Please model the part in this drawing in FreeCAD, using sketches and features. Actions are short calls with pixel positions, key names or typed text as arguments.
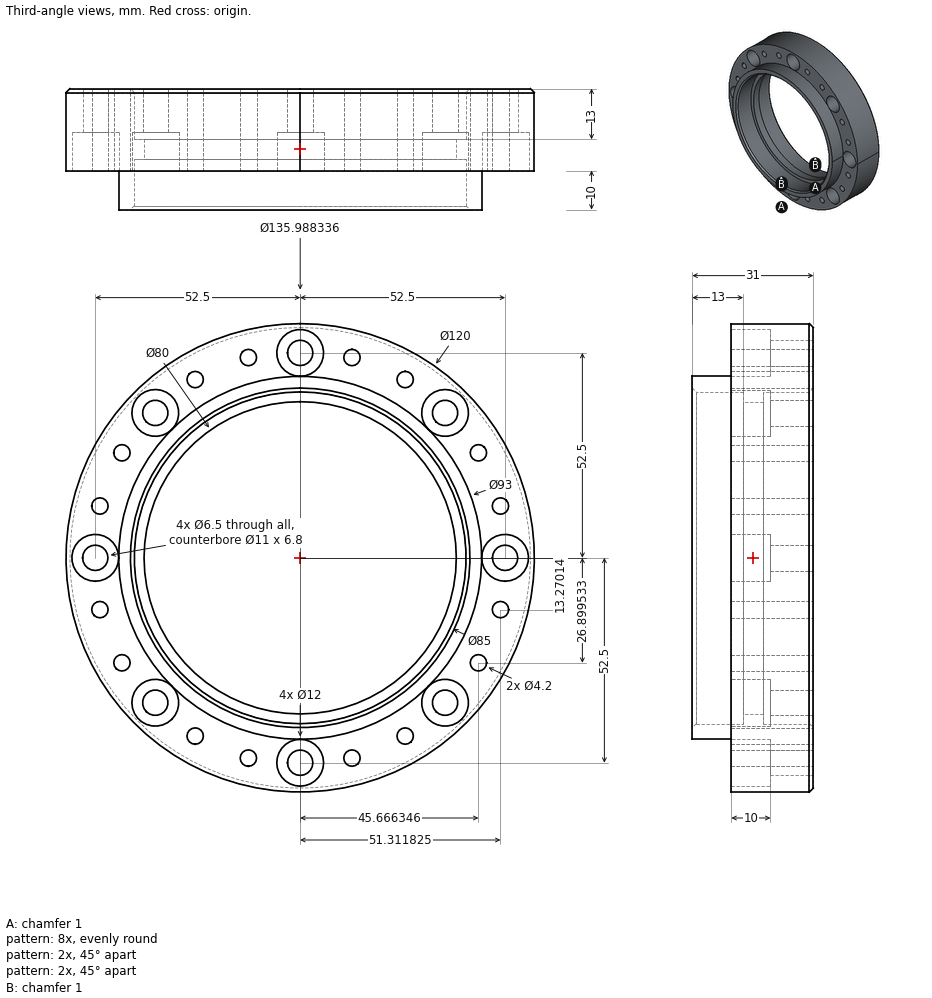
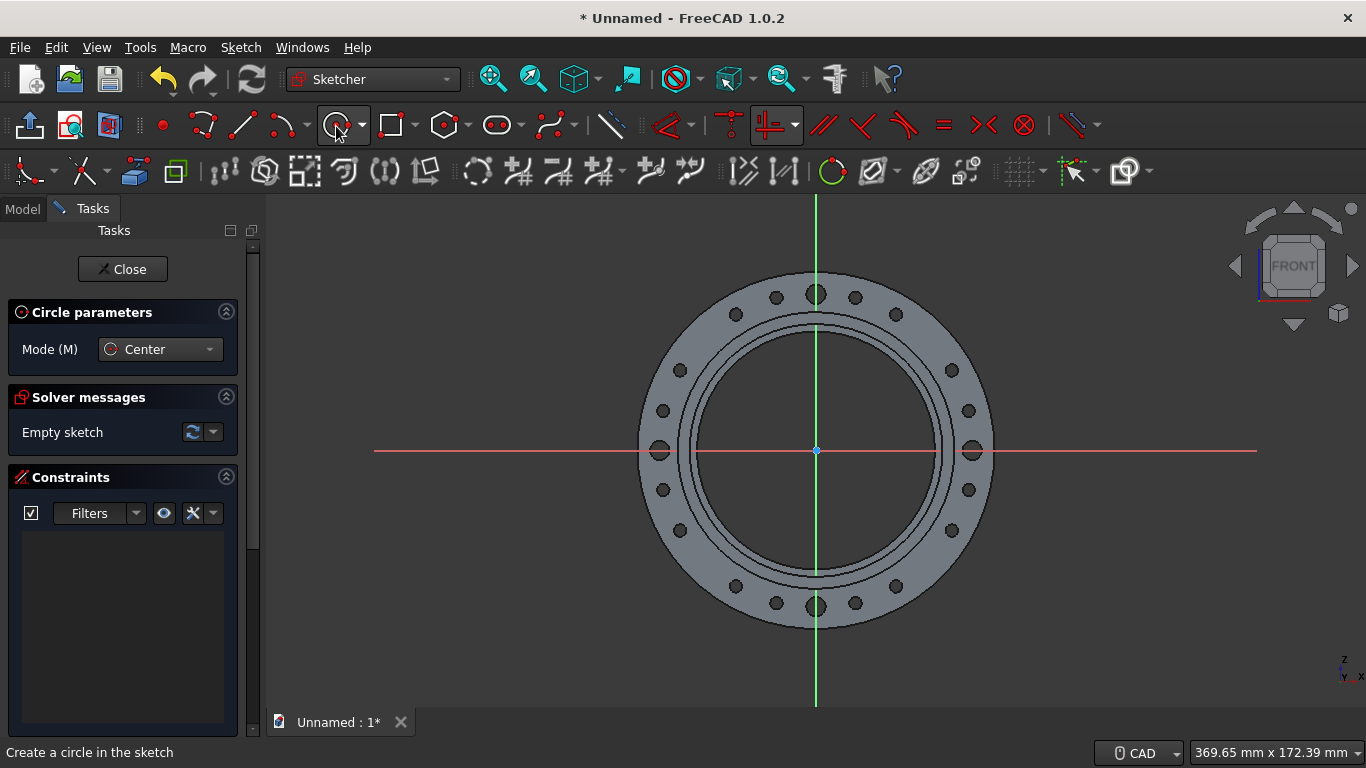
scroll(816, 607, up, 2)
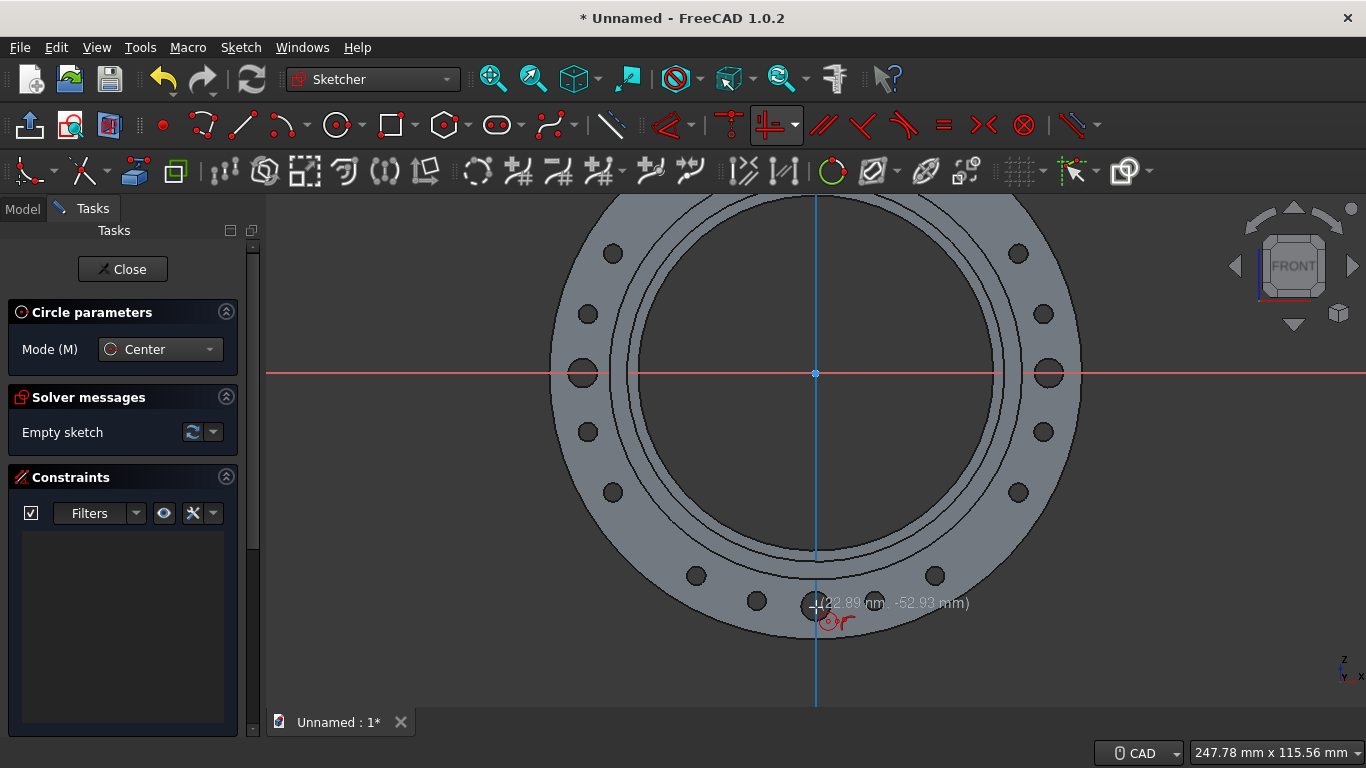
click(816, 606)
move(835, 587)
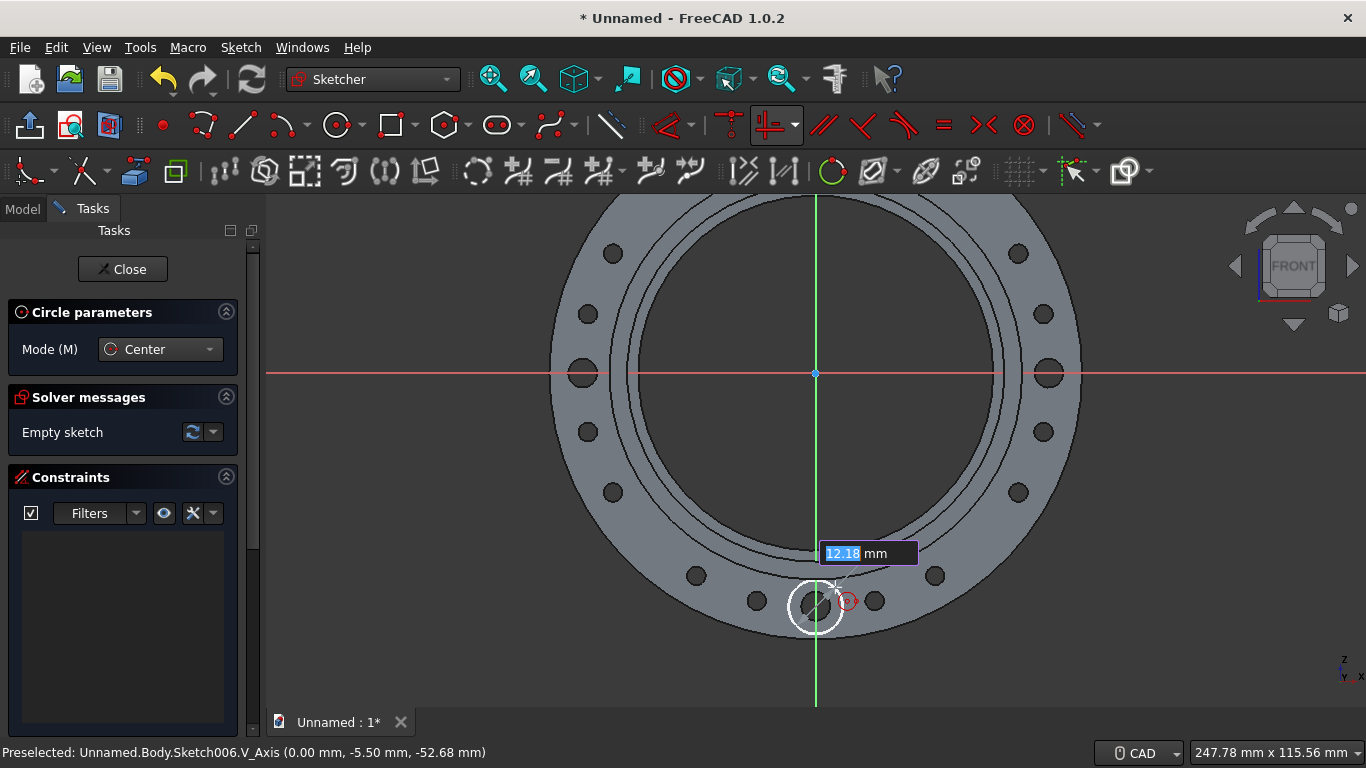
text(12)
key(Return)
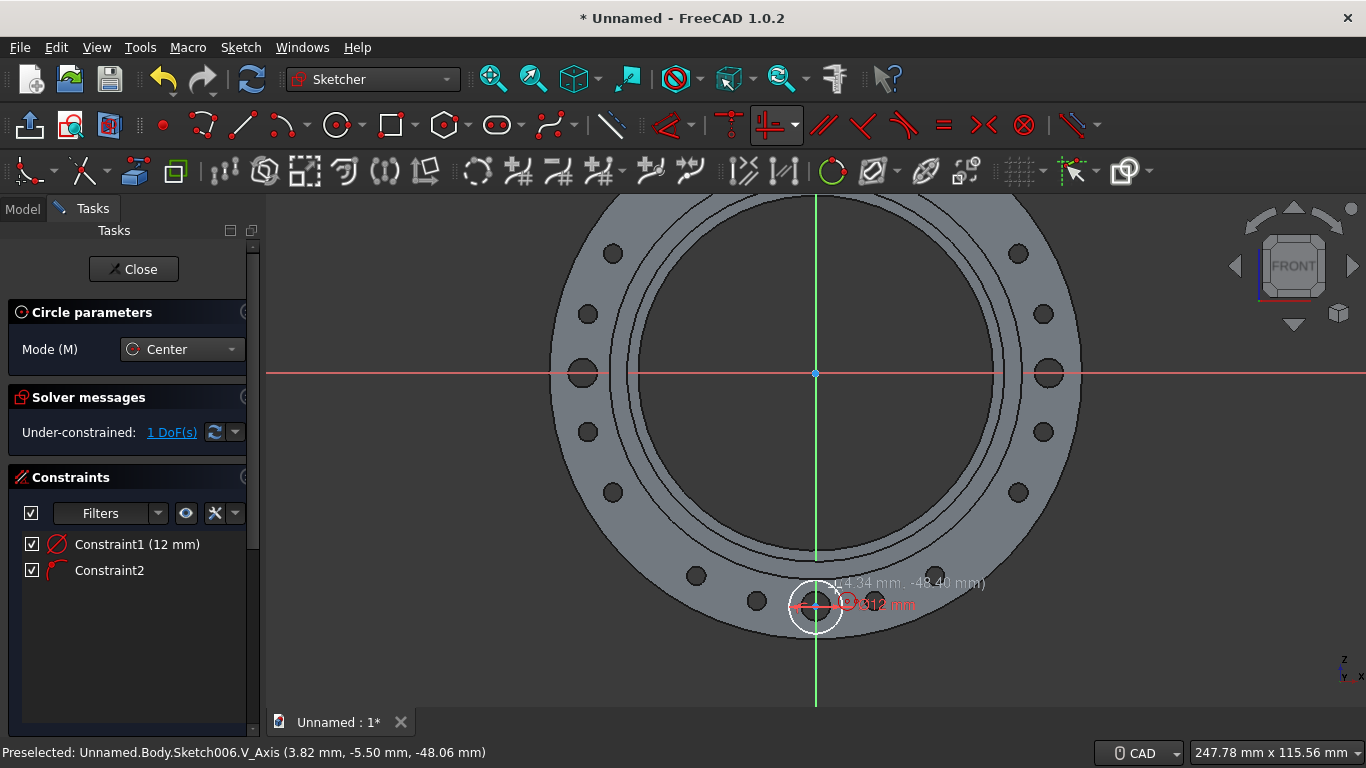
click(1049, 373)
move(1068, 354)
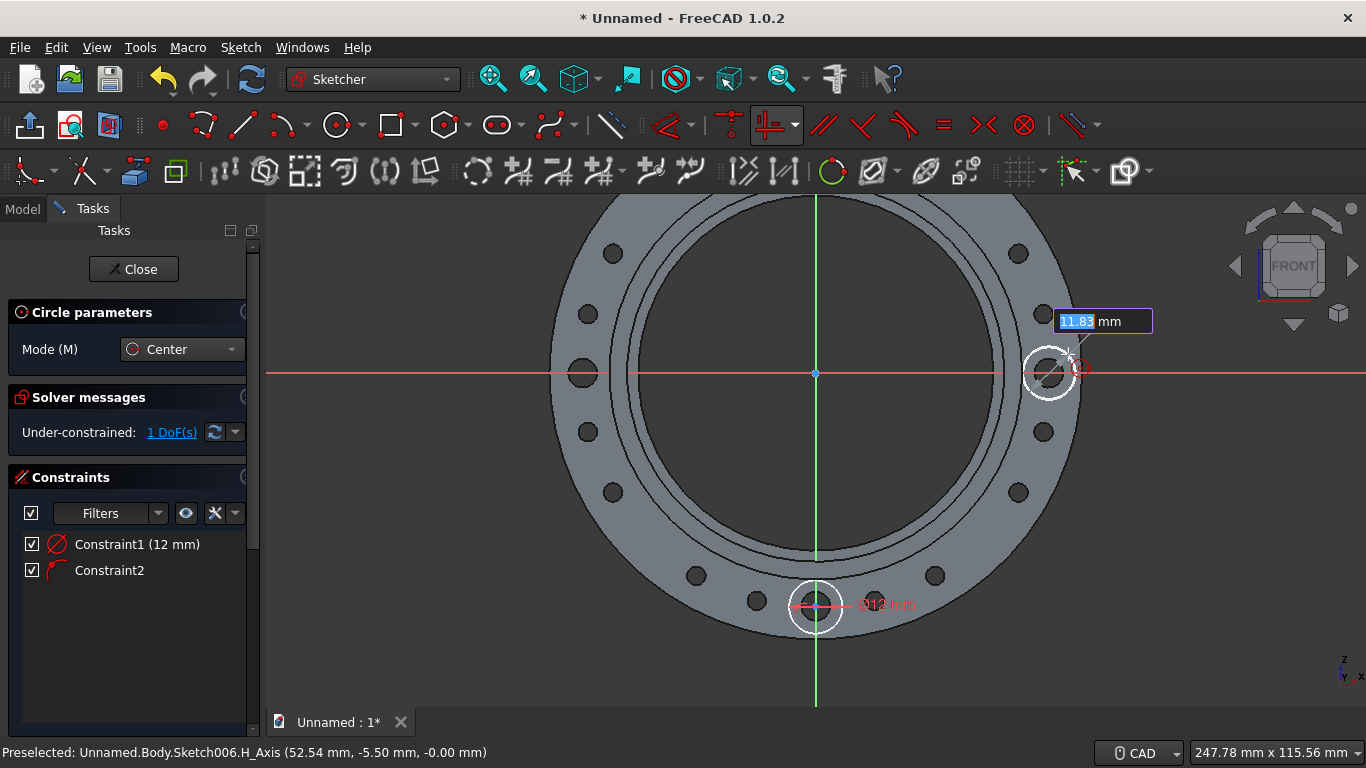
text(12)
key(Return)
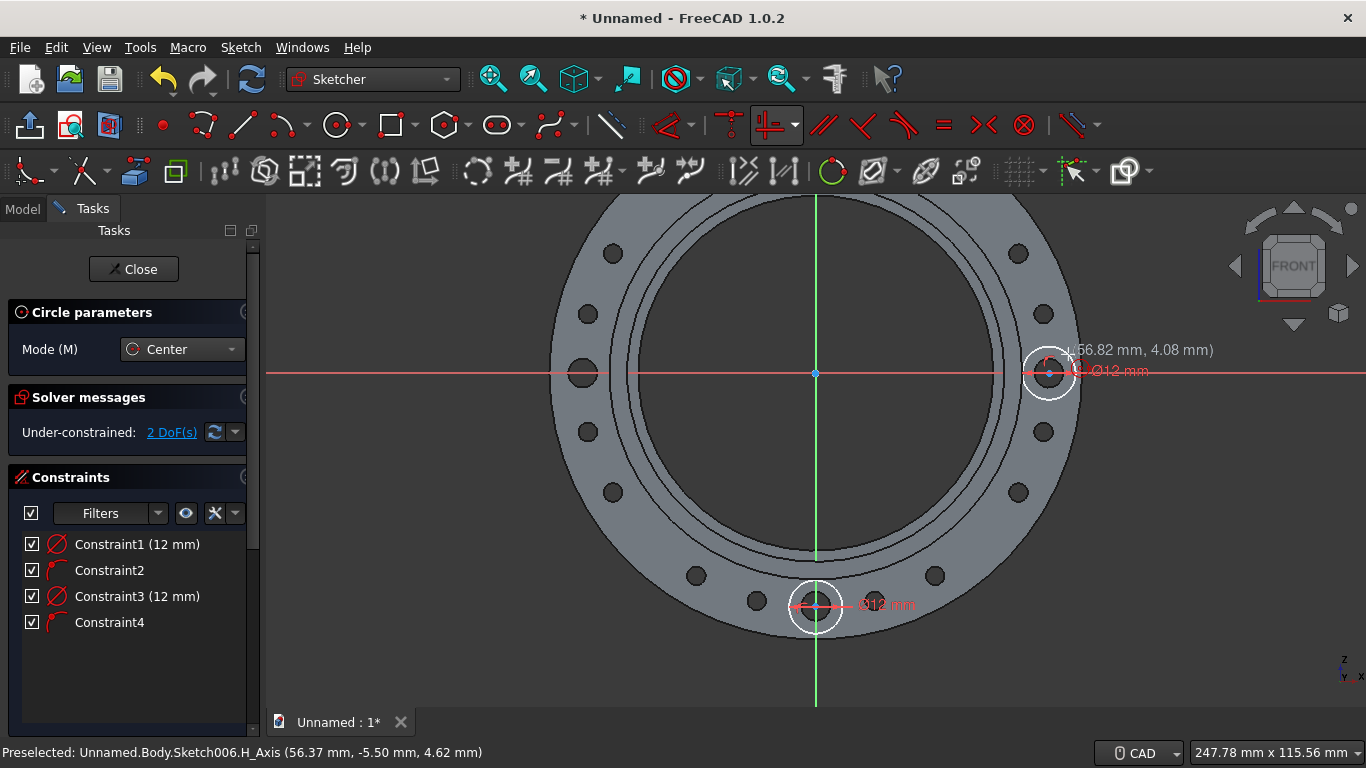
scroll(609, 608, down, 2)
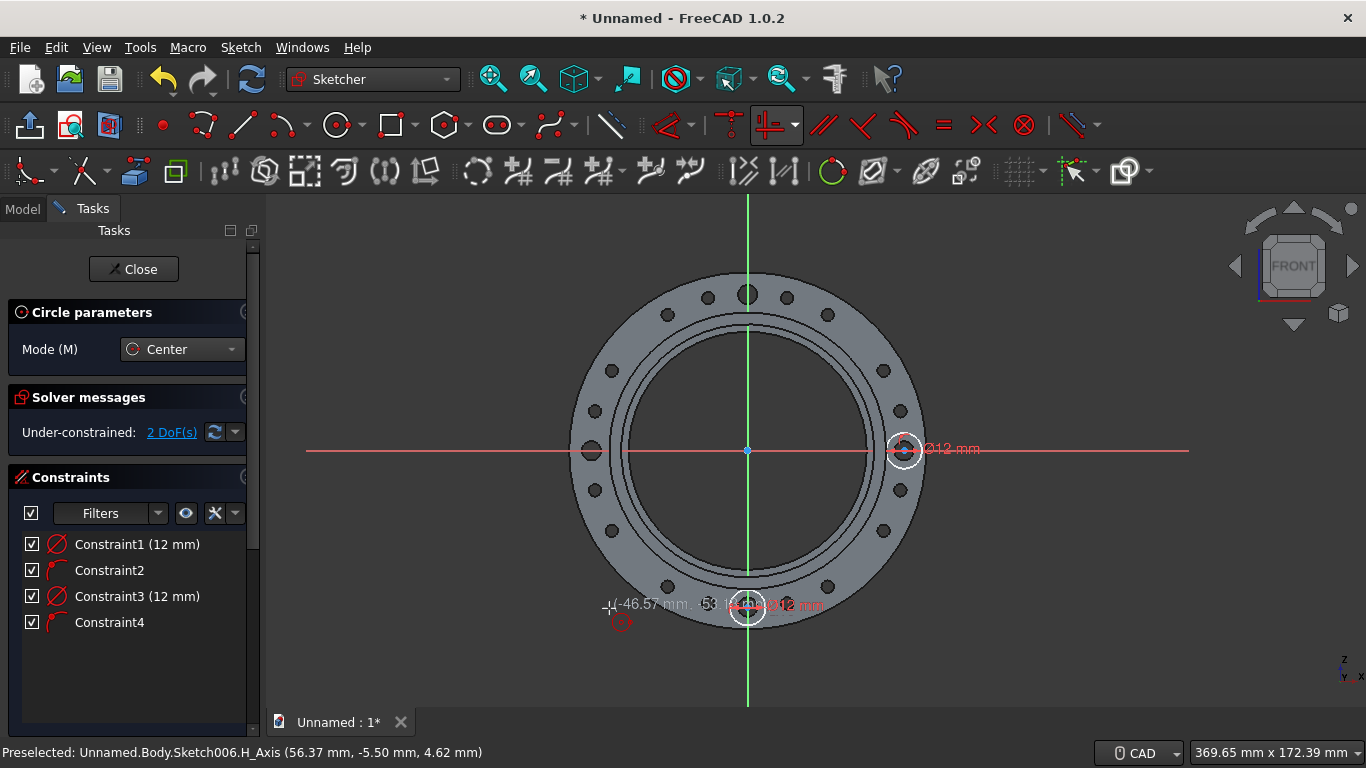
scroll(748, 295, up, 2)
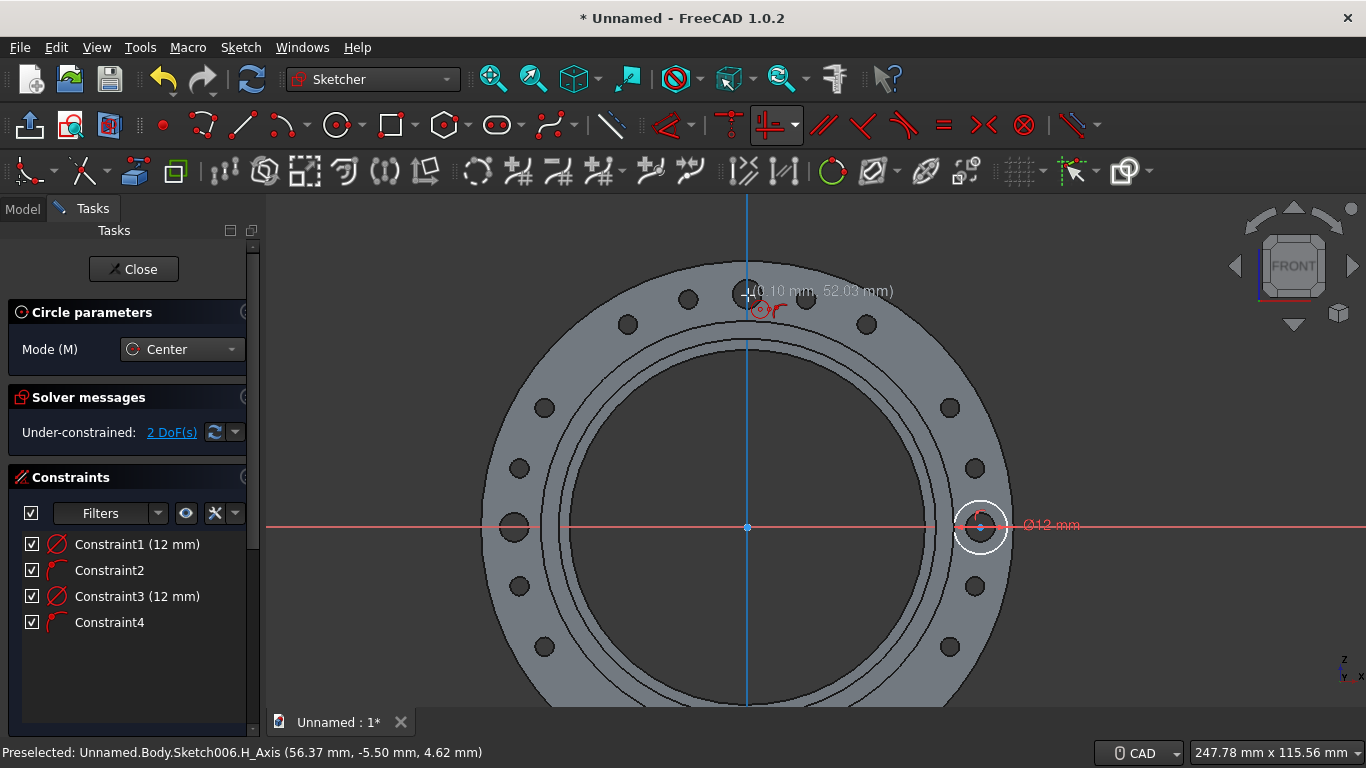
click(747, 294)
move(766, 275)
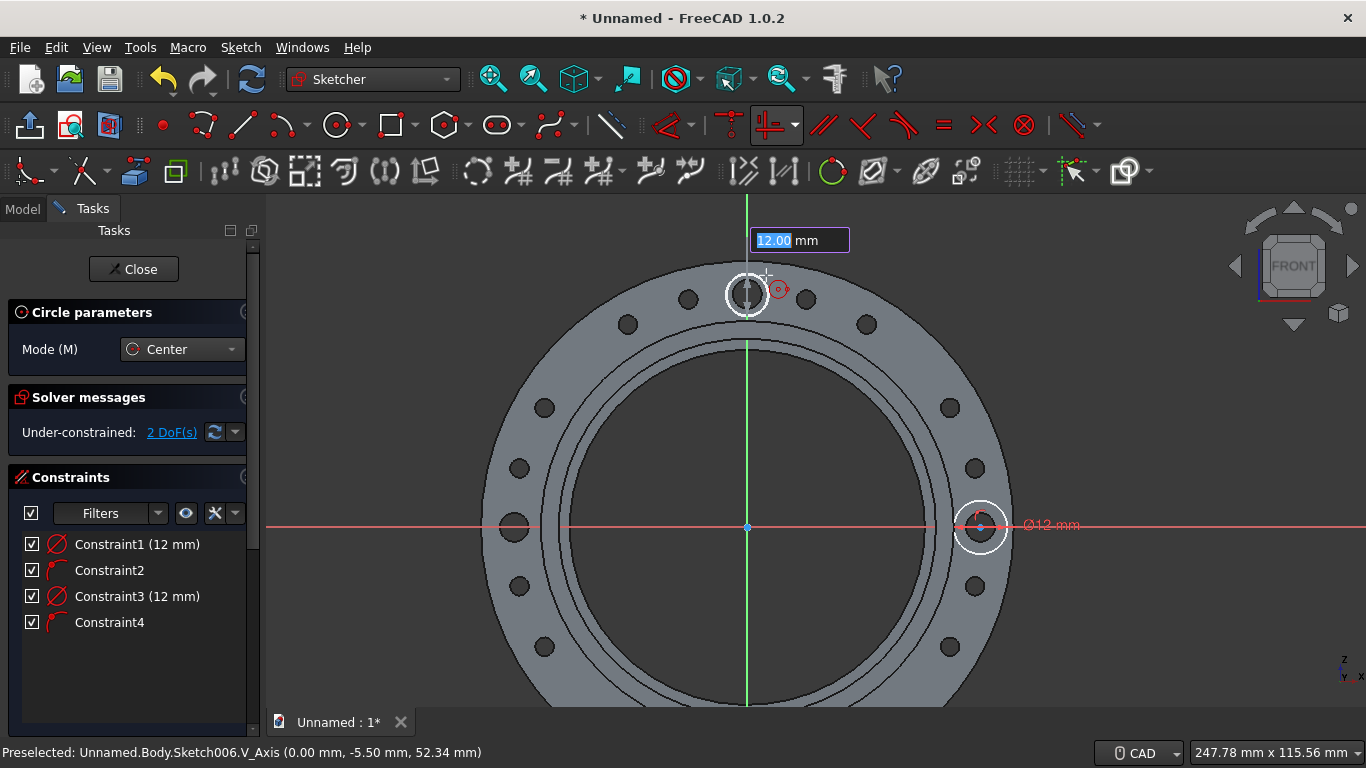
text(12)
key(Return)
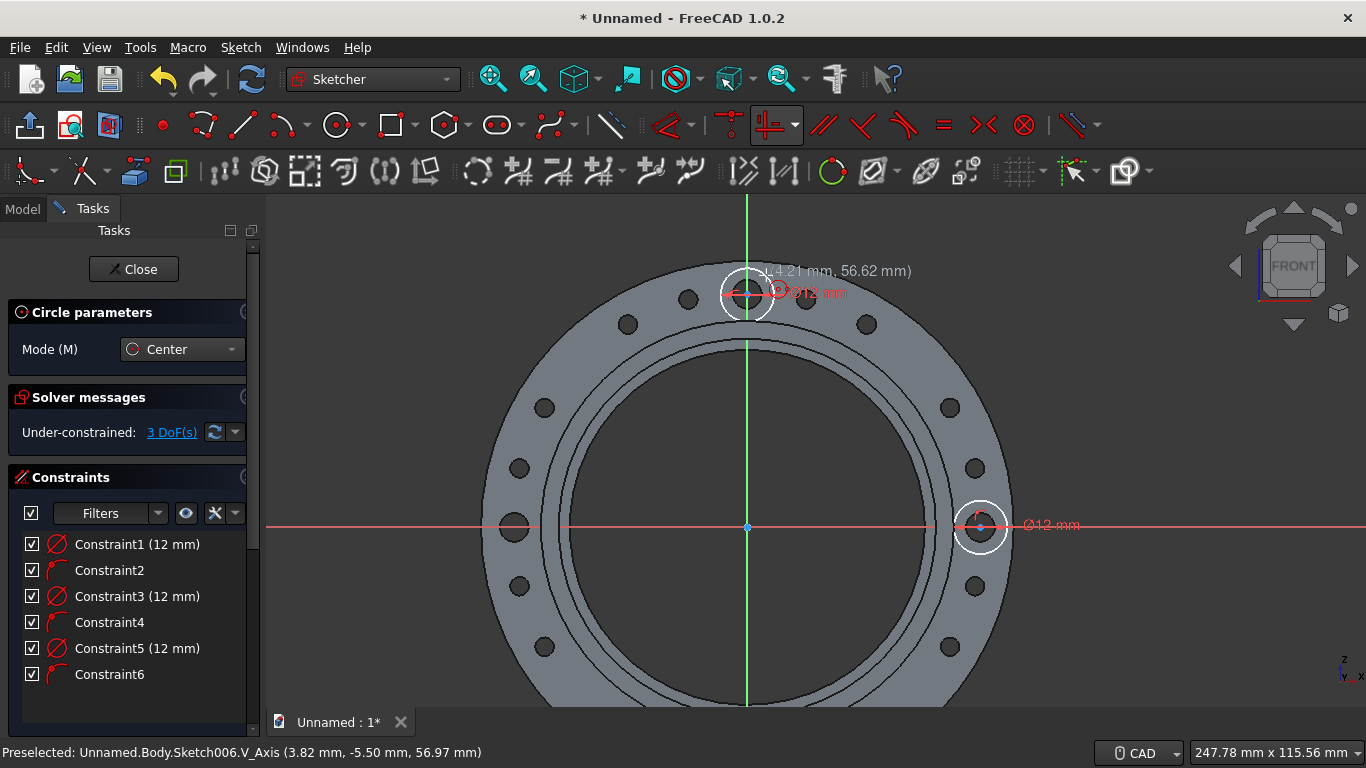
click(514, 527)
move(533, 509)